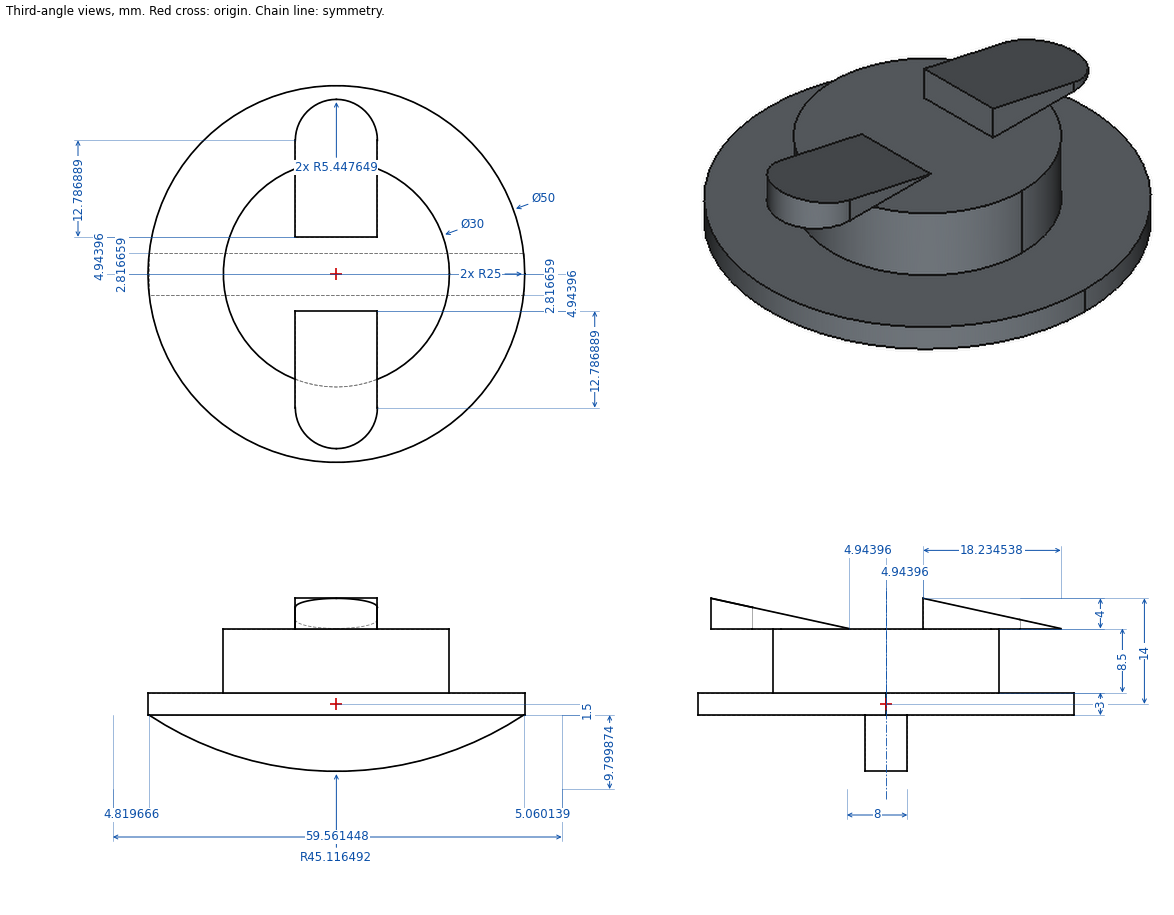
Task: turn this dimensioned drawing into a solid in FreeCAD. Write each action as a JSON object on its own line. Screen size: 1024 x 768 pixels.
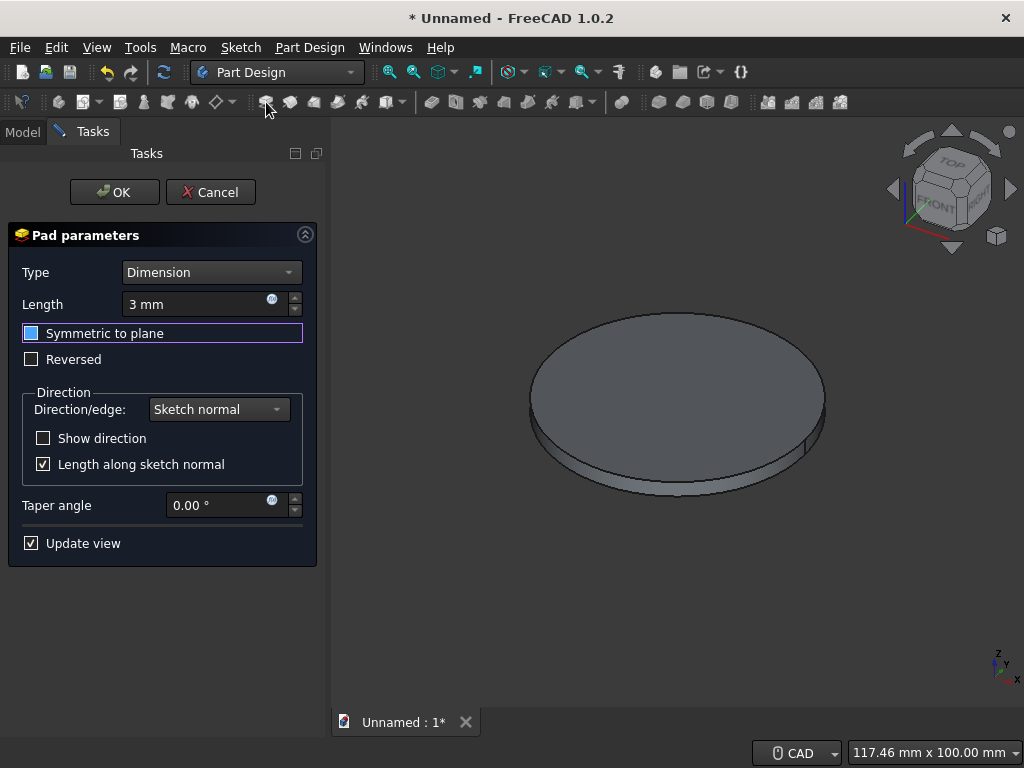
{"action": "left_click", "coordinate": [30, 333]}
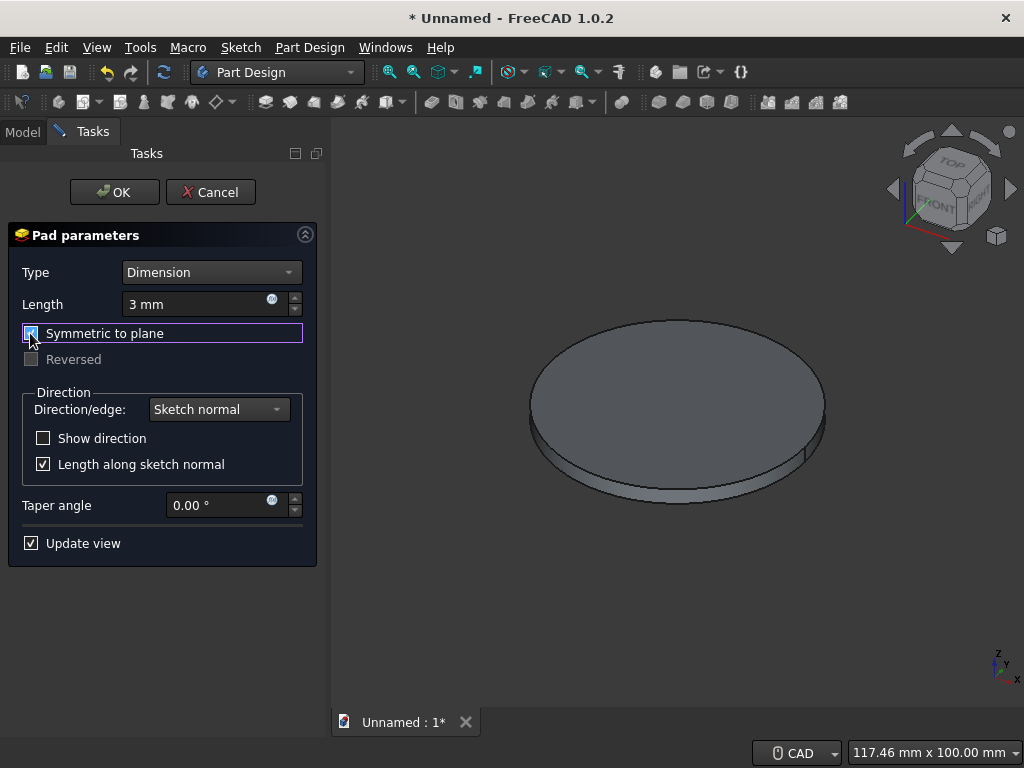
{"action": "left_click", "coordinate": [115, 192]}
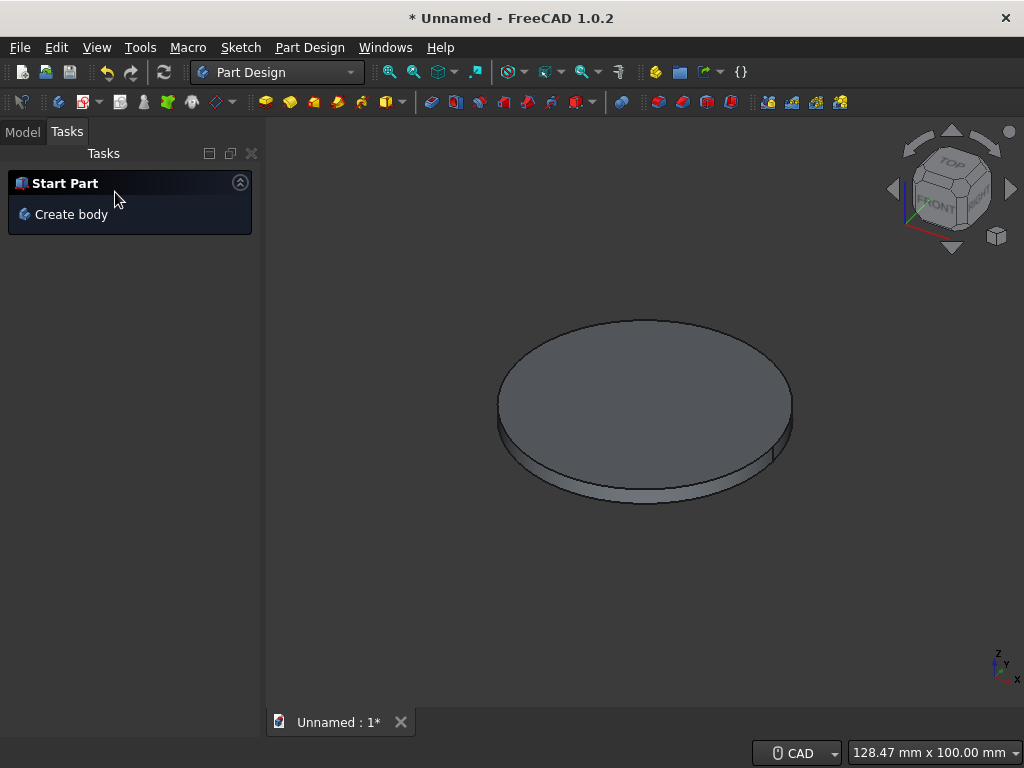
{"action": "key", "text": "5"}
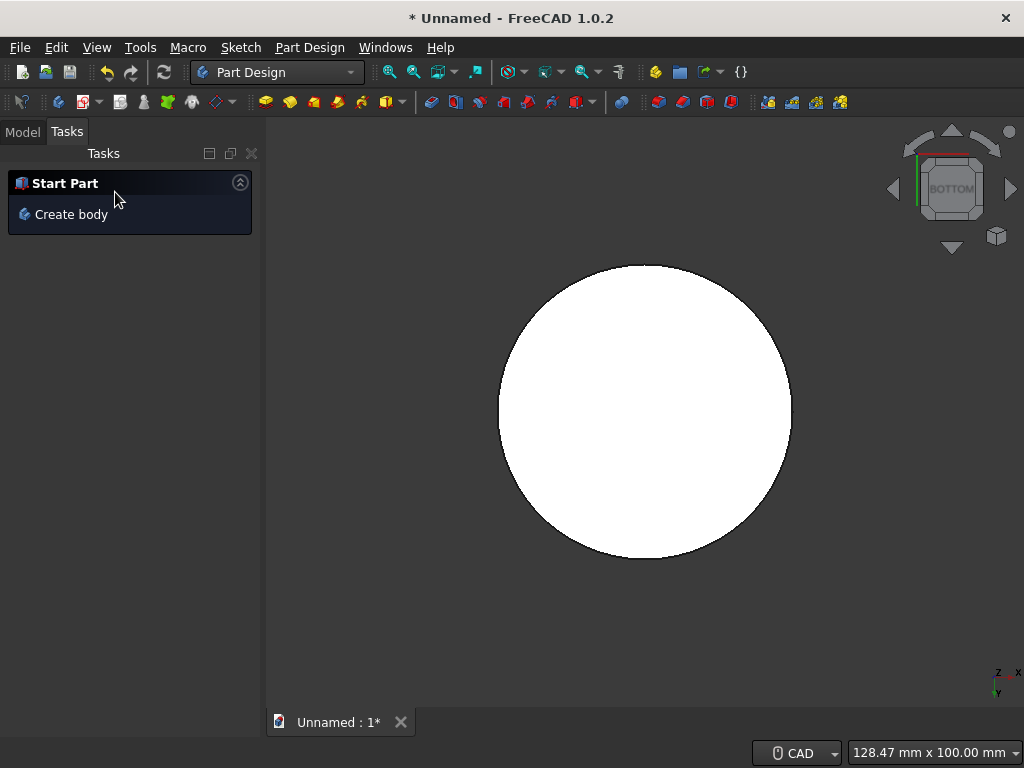
{"action": "left_click", "coordinate": [645, 411]}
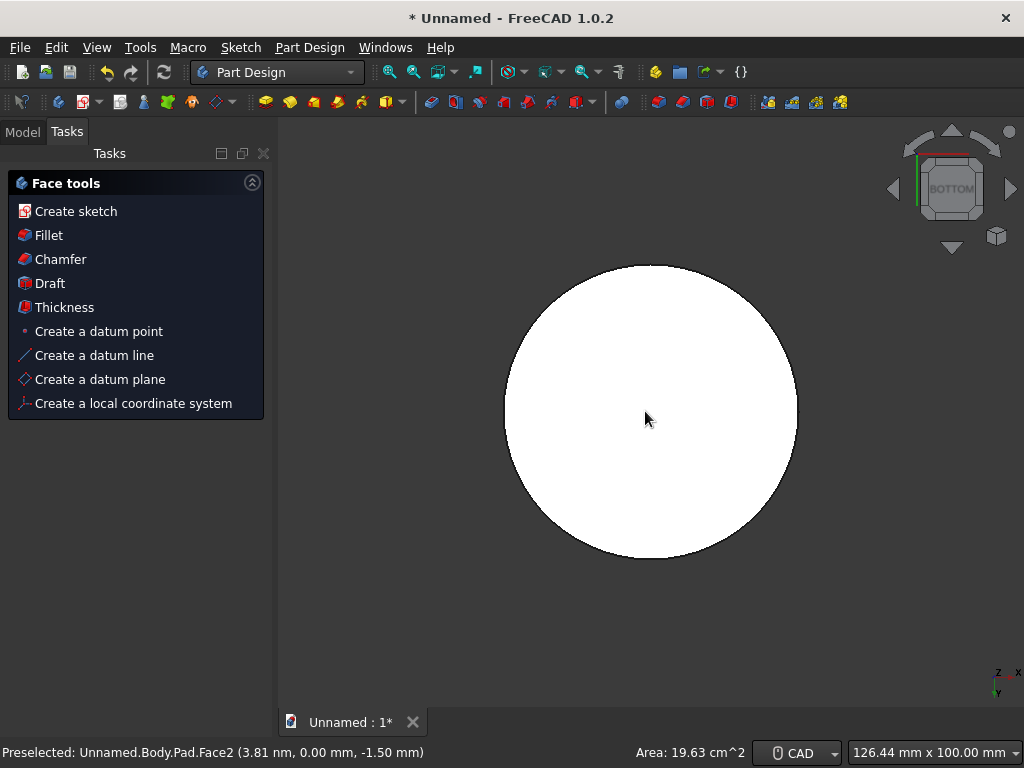
{"action": "left_click", "coordinate": [84, 102]}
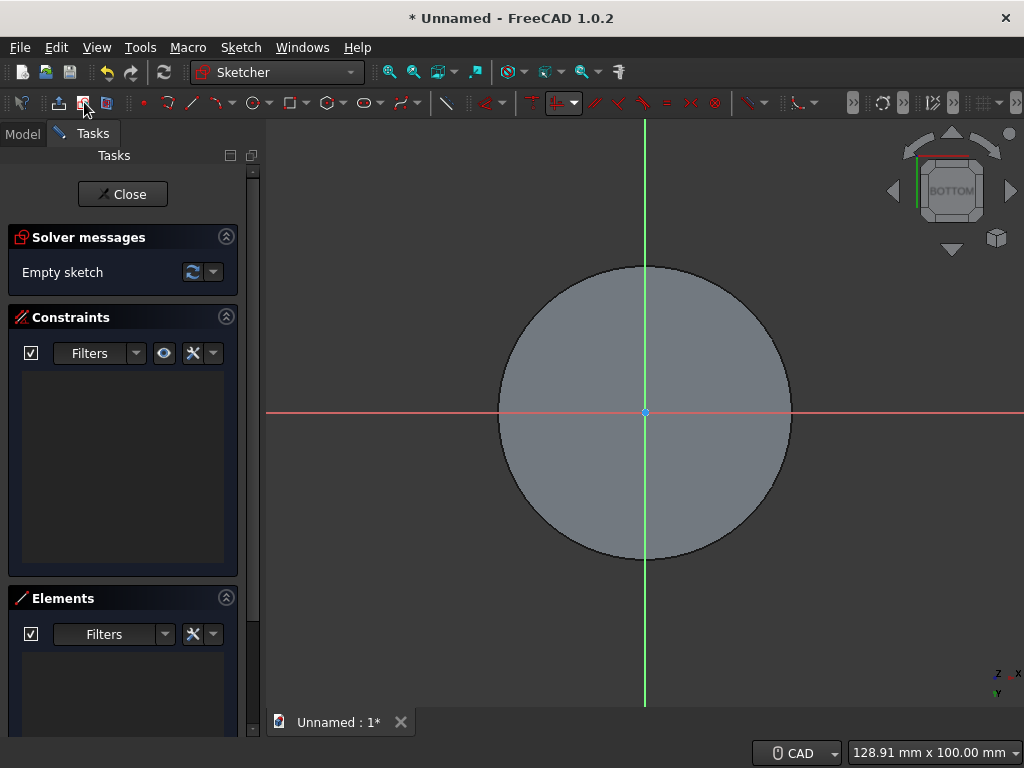
{"action": "scroll", "coordinate": [784, 413], "scroll_direction": "up", "scroll_amount": 2}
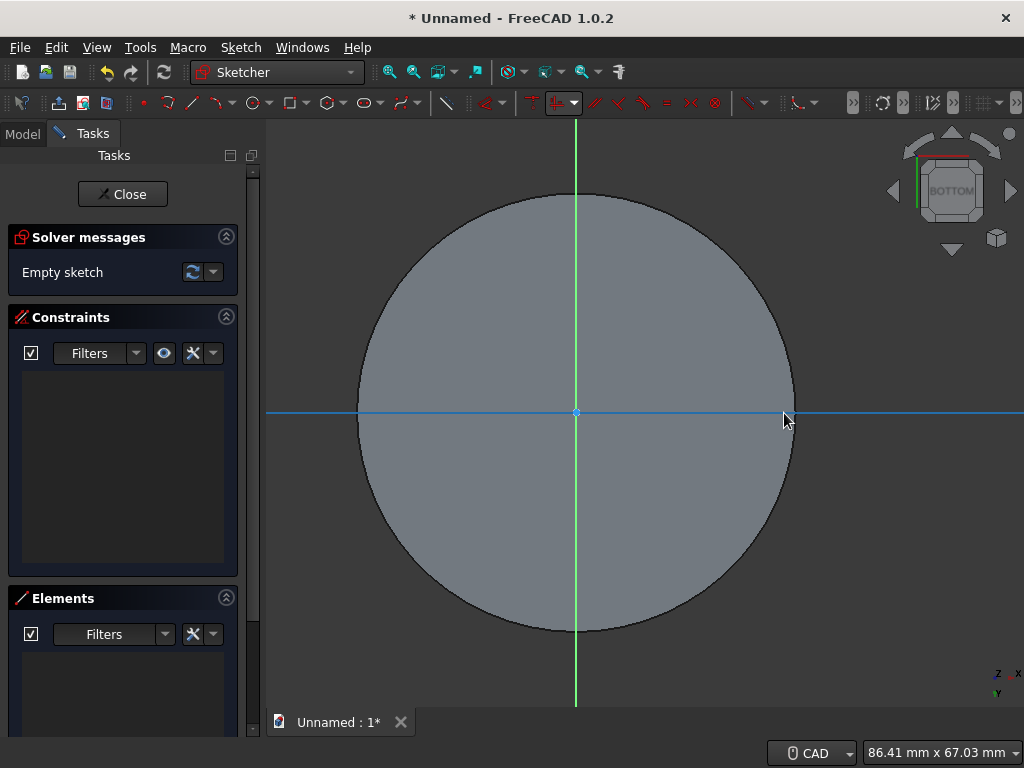
{"action": "left_click", "coordinate": [192, 104]}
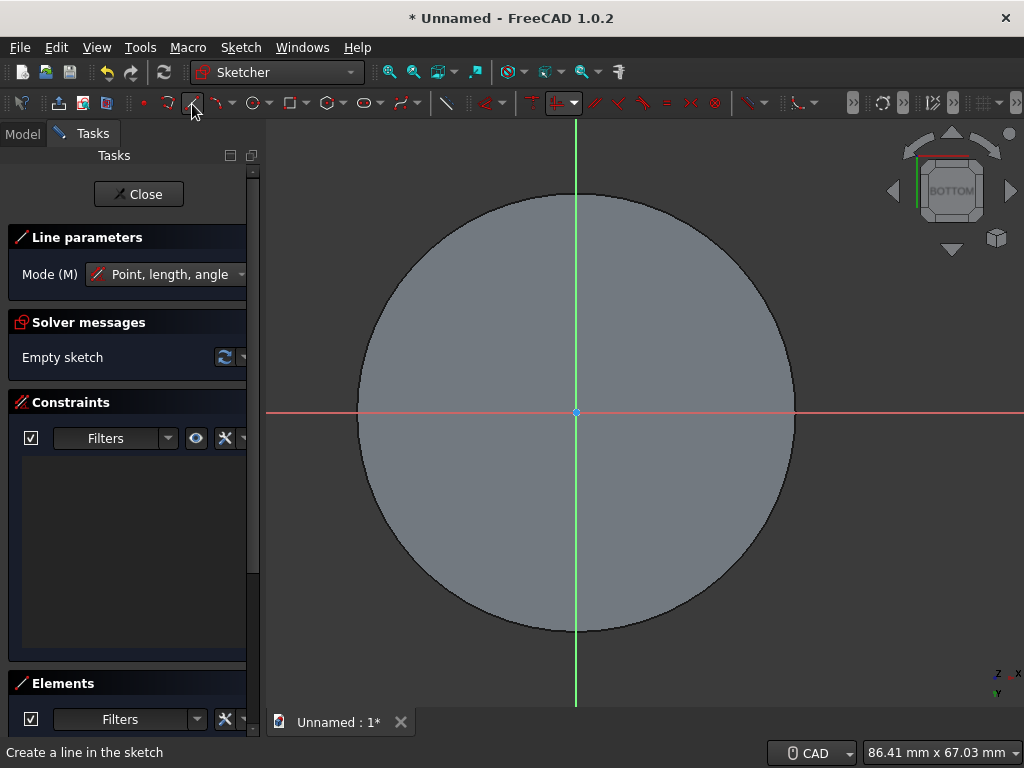
{"action": "left_click", "coordinate": [358, 437]}
{"action": "left_click", "coordinate": [794, 437]}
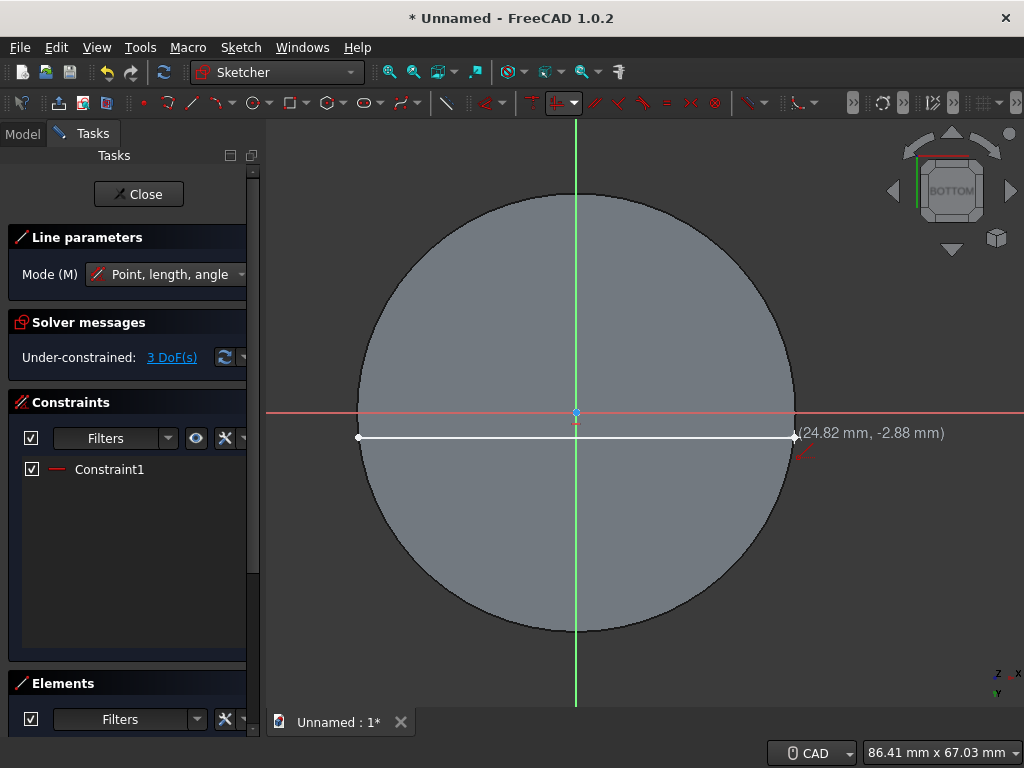
{"action": "left_click", "coordinate": [794, 388]}
{"action": "left_click", "coordinate": [358, 388]}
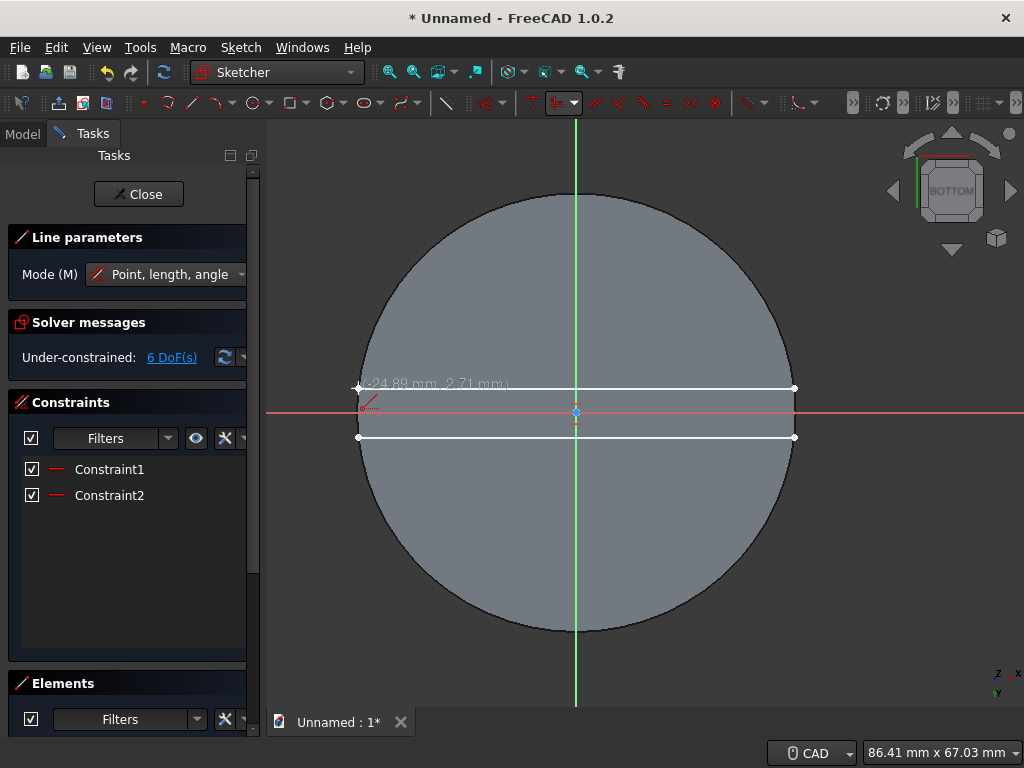
{"action": "left_click", "coordinate": [216, 104]}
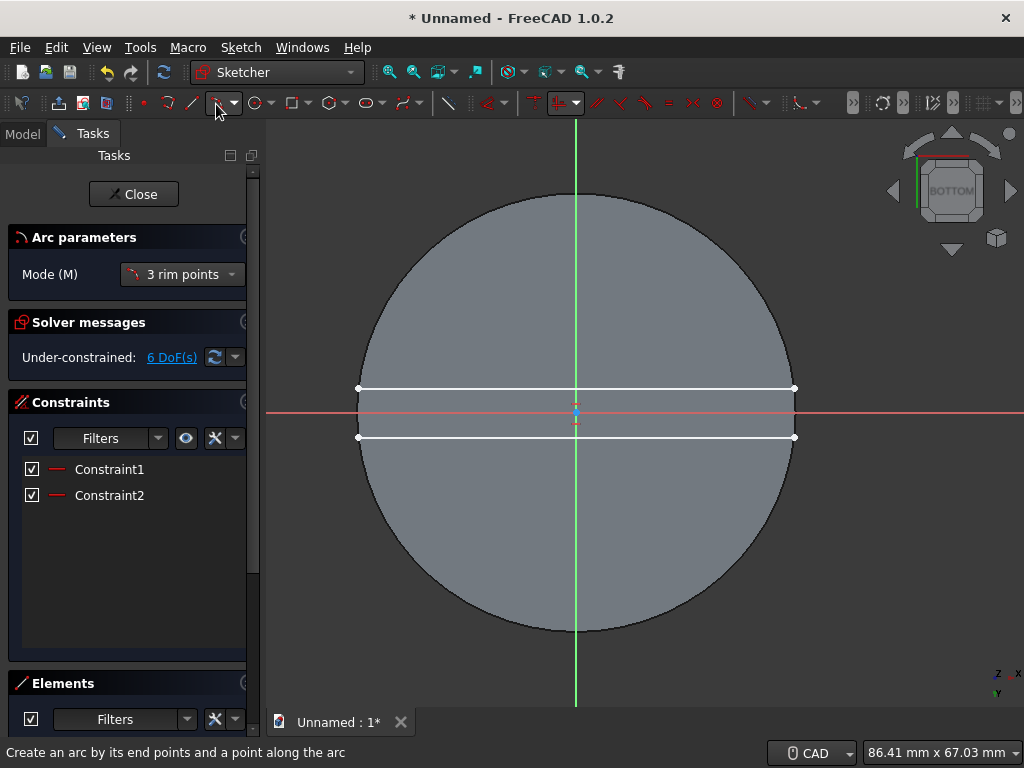
{"action": "left_click", "coordinate": [794, 438]}
{"action": "left_click", "coordinate": [794, 389]}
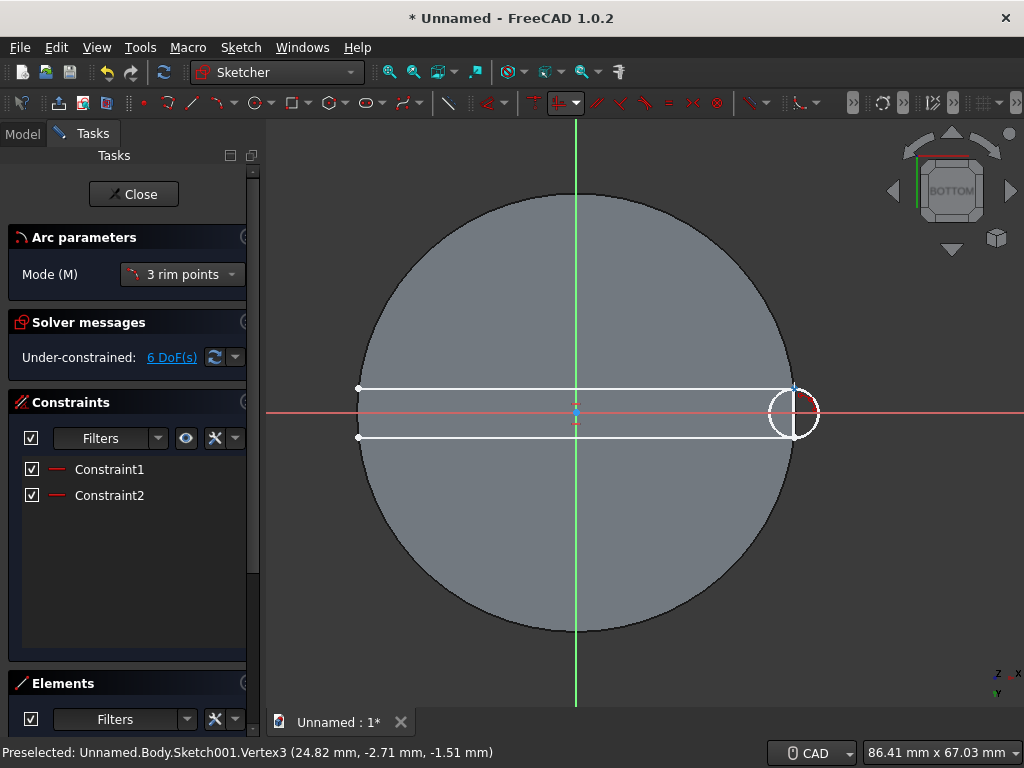
{"action": "scroll", "coordinate": [796, 418], "scroll_direction": "up", "scroll_amount": 13}